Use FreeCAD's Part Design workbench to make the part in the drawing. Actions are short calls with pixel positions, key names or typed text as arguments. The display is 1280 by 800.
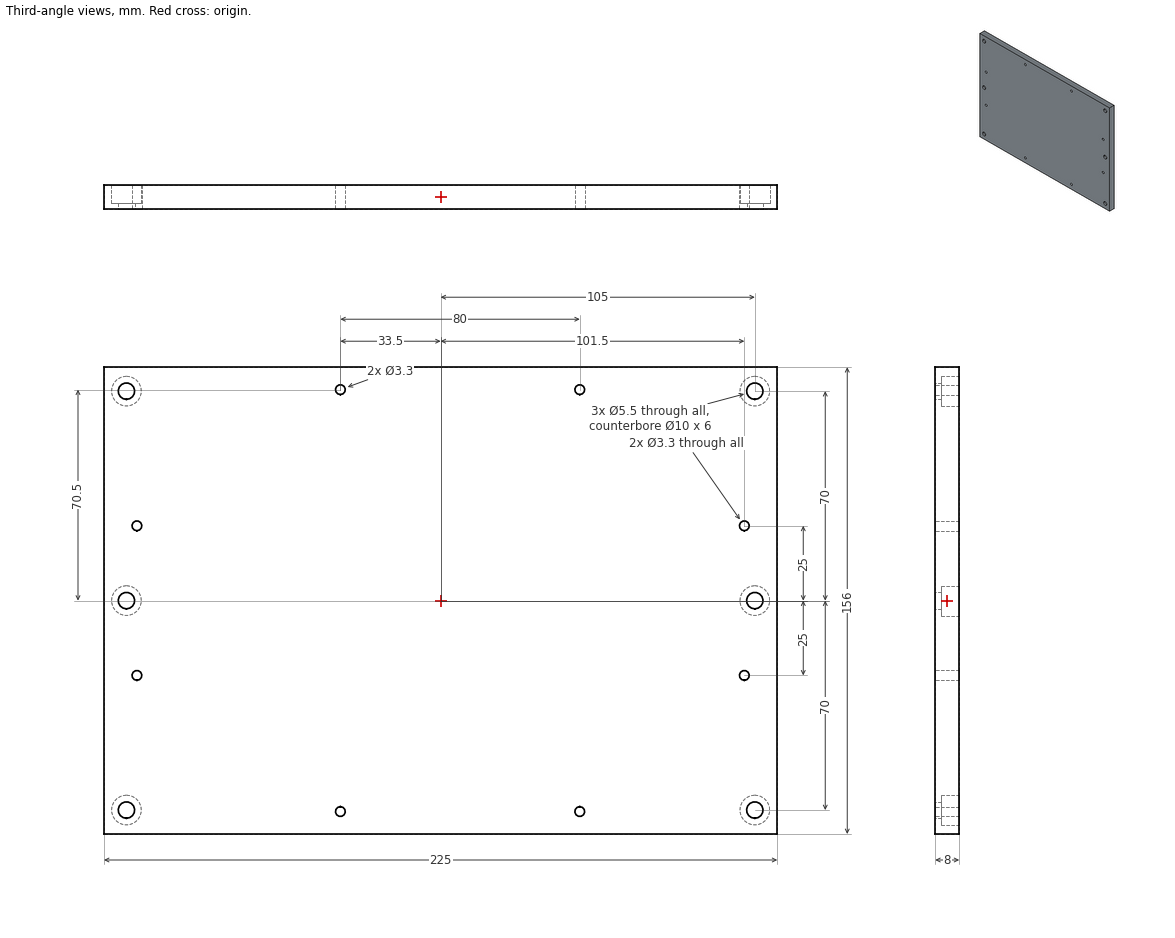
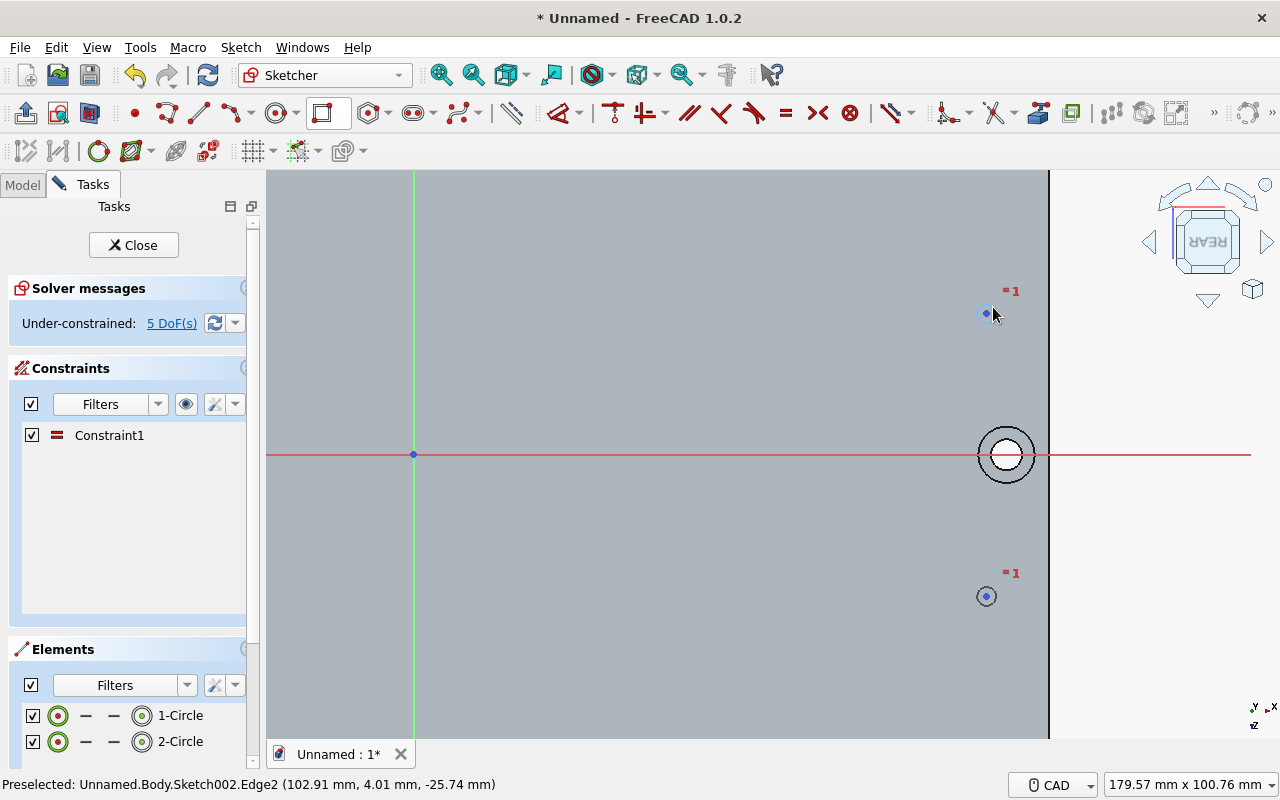
click(987, 596)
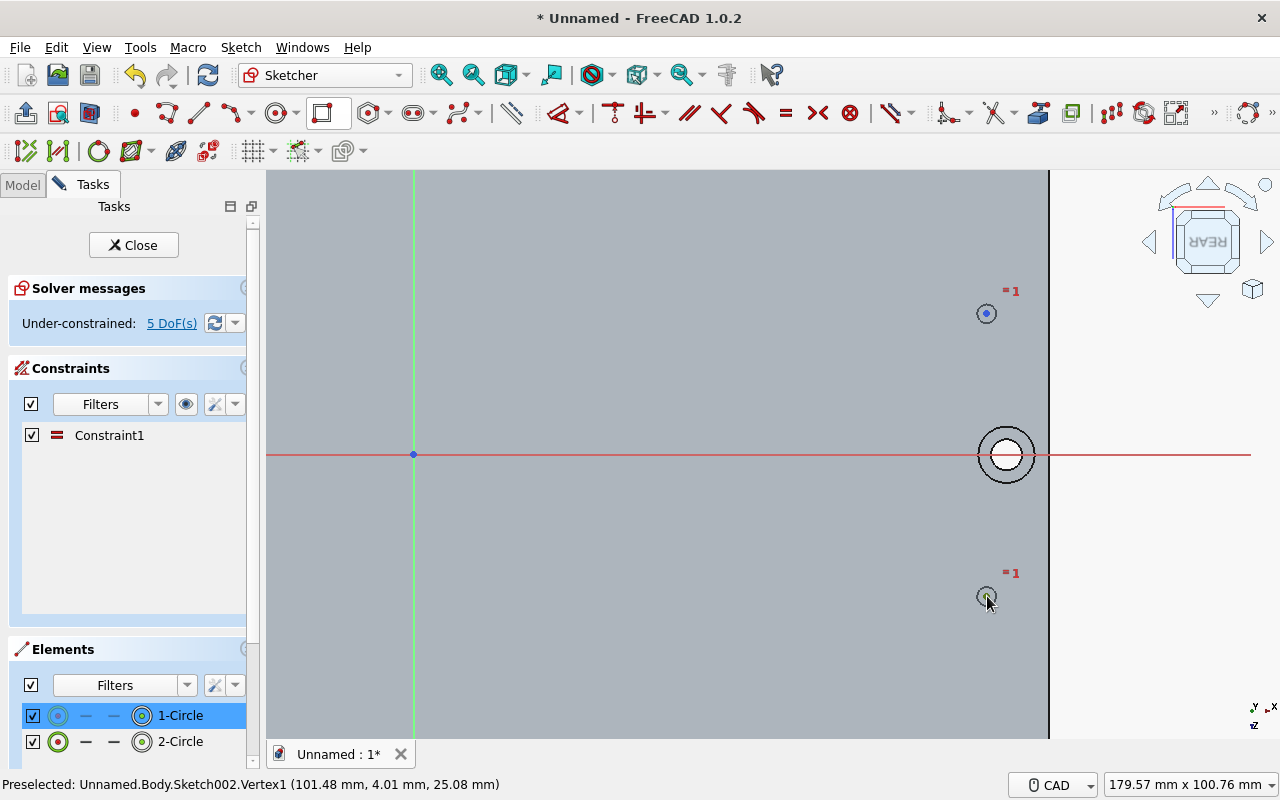
click(987, 314)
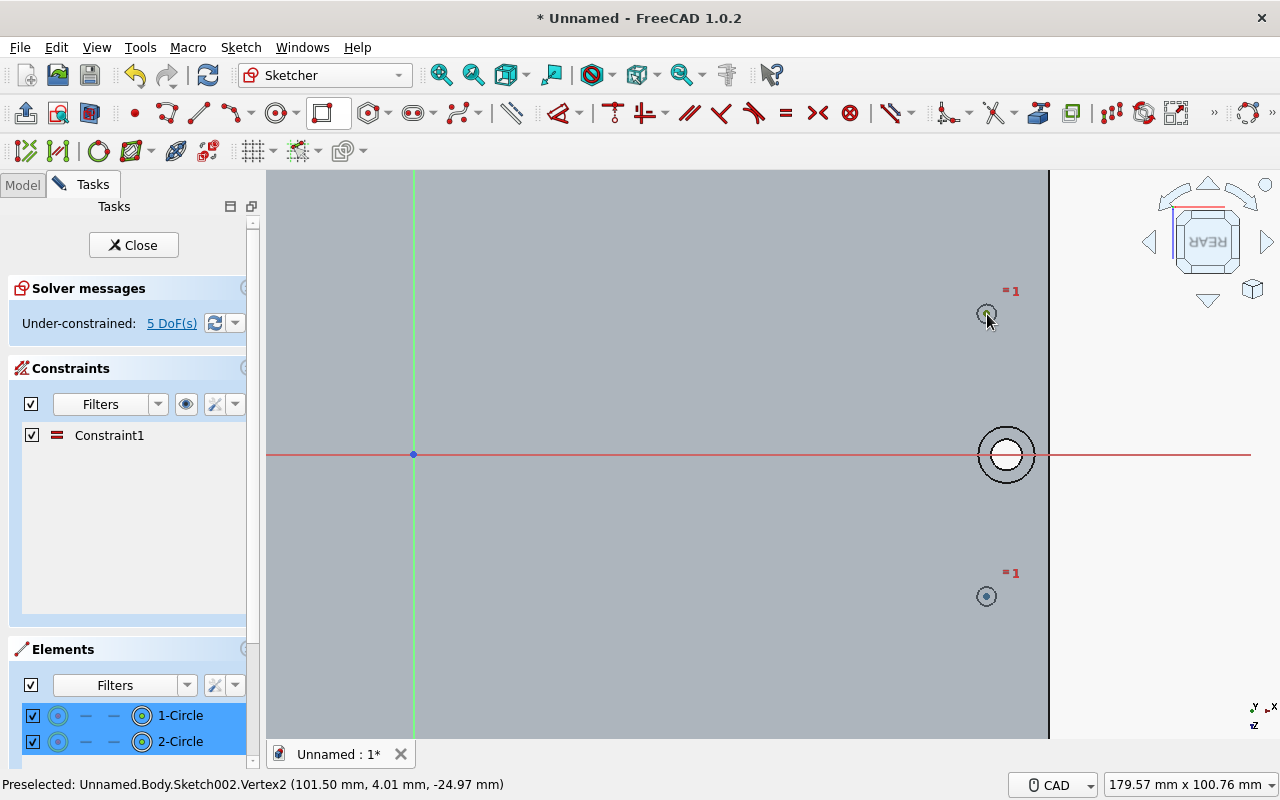
key(v)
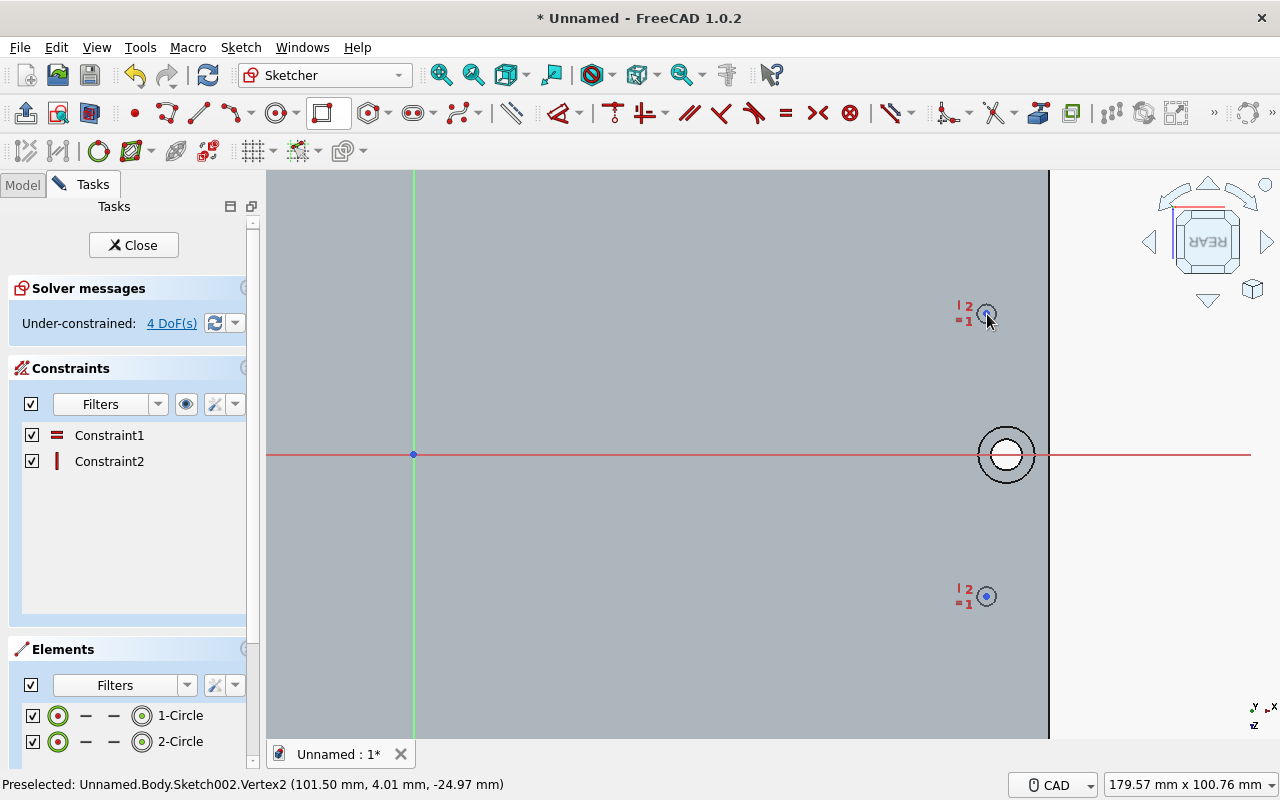
key(d)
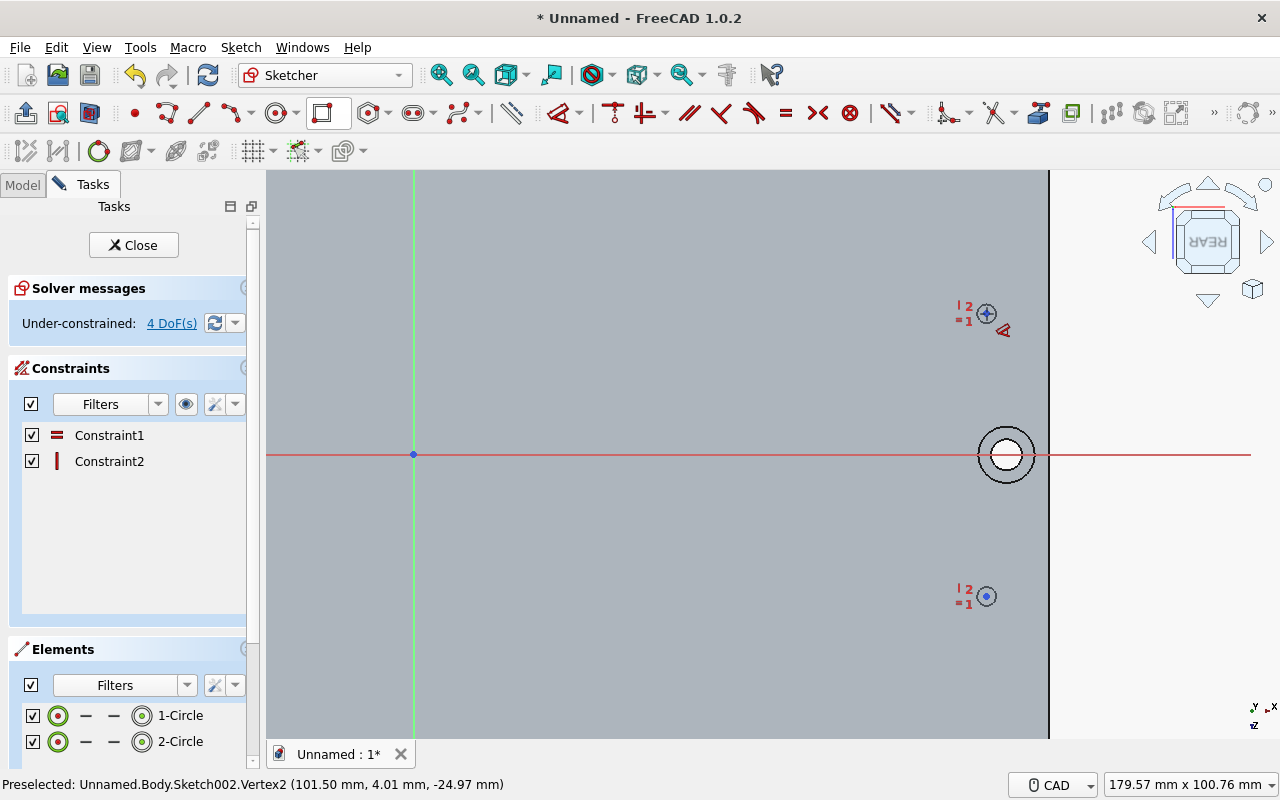
scroll(993, 590, up, 4)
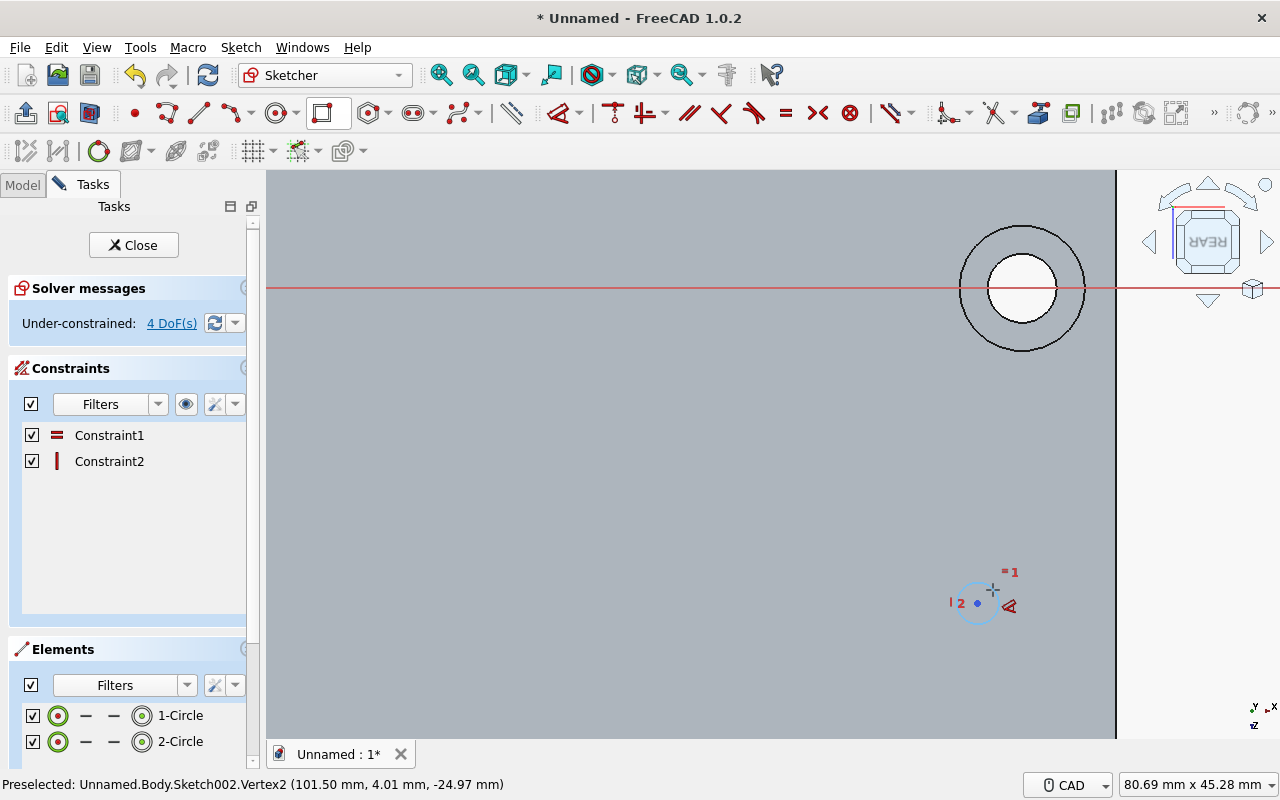
click(993, 589)
click(1016, 567)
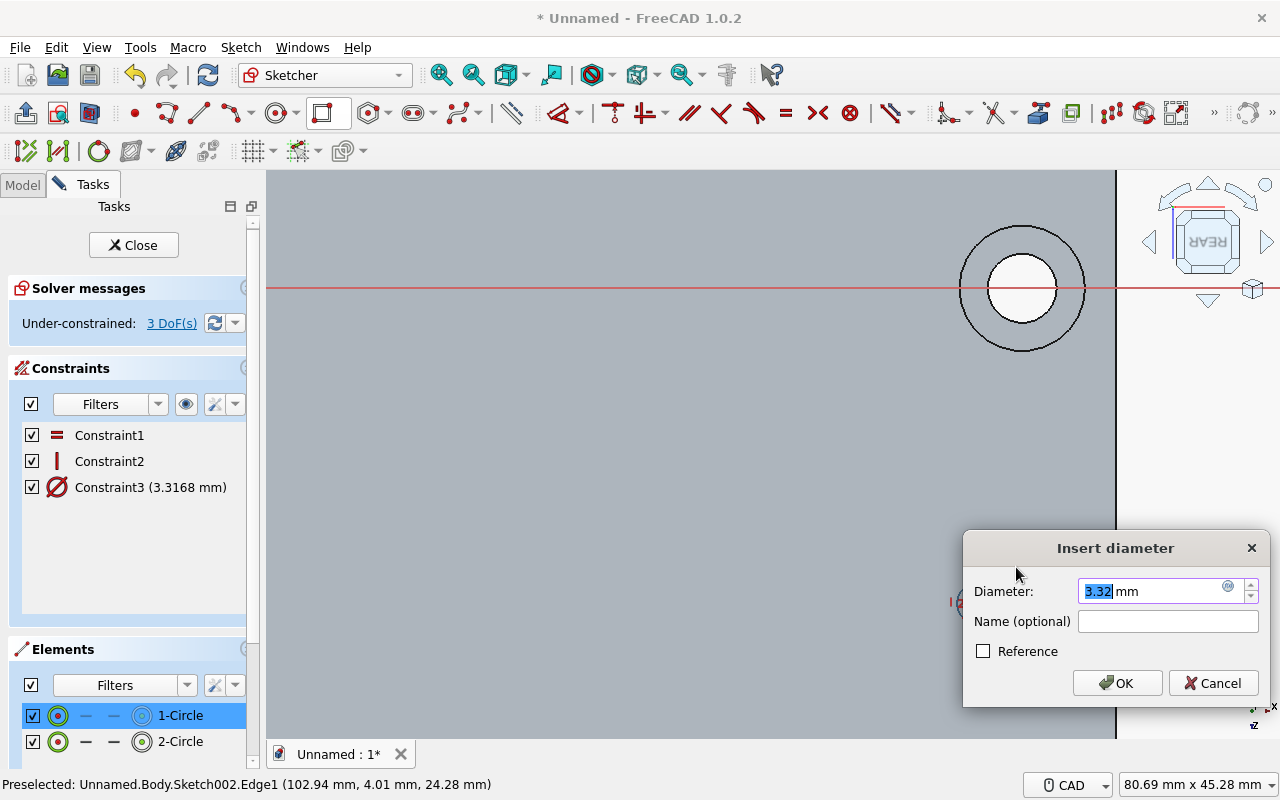
text(3.3)
key(Return)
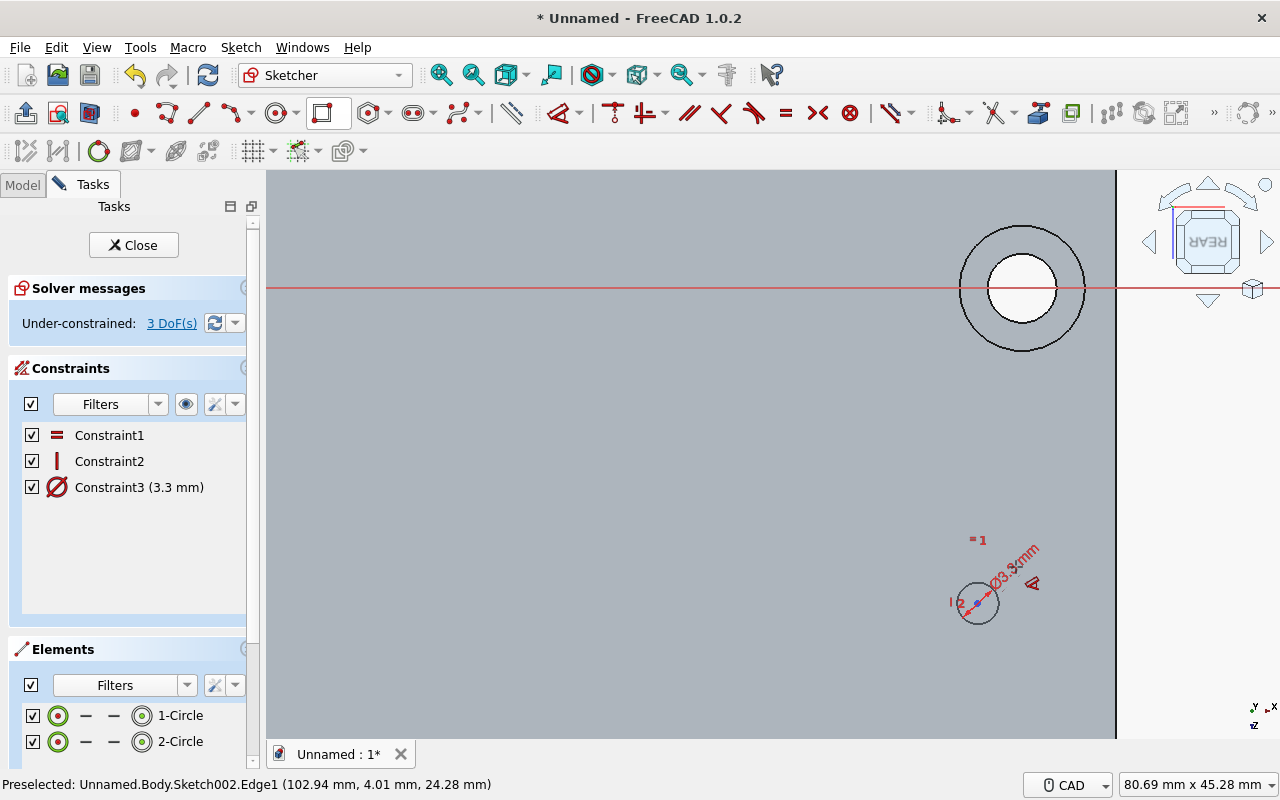
click(978, 603)
click(1012, 446)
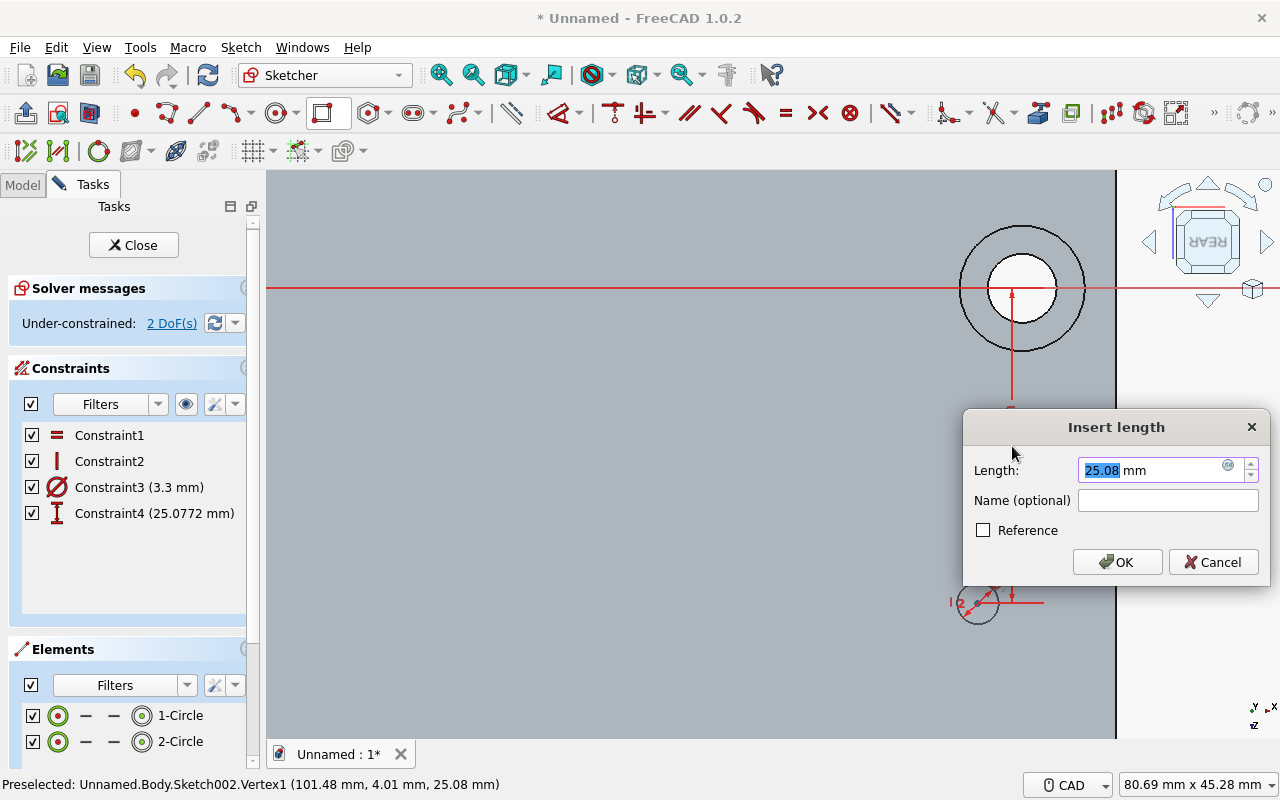
text(25)
key(Return)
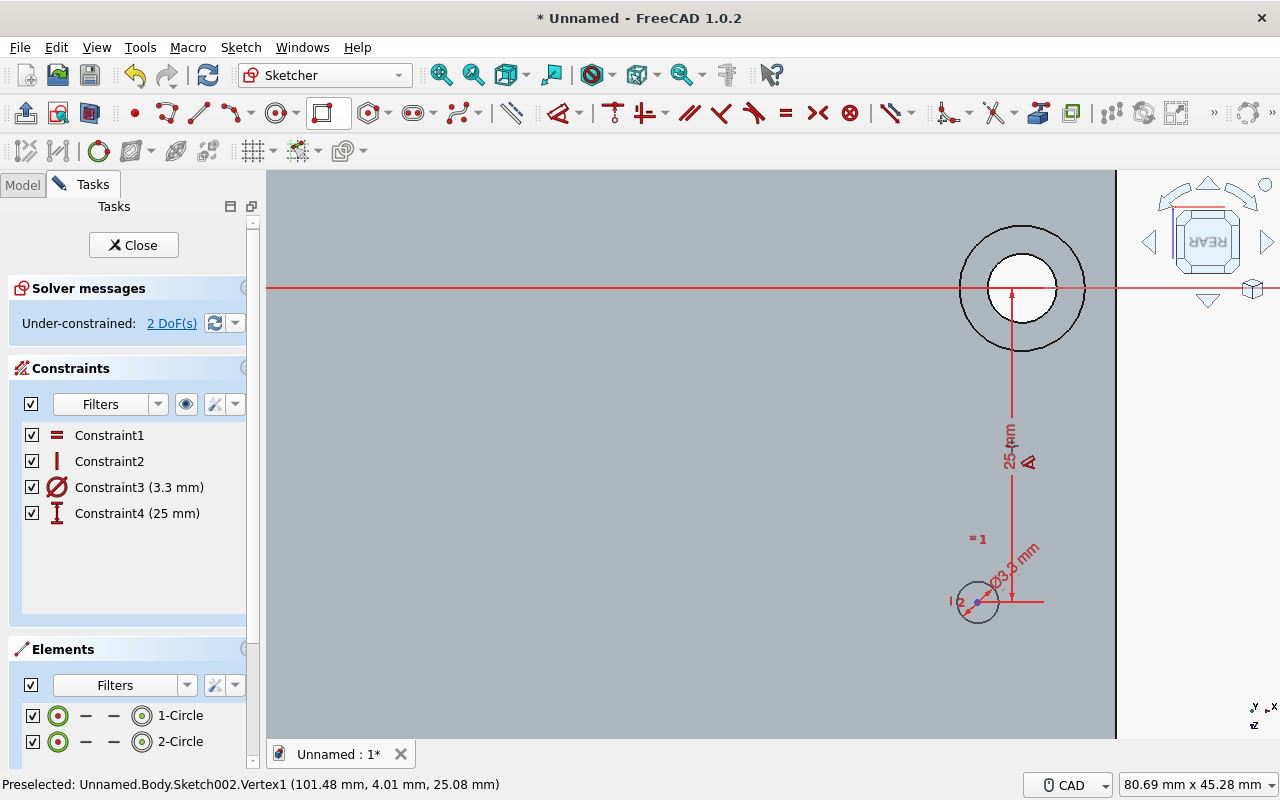
scroll(993, 590, down, 4)